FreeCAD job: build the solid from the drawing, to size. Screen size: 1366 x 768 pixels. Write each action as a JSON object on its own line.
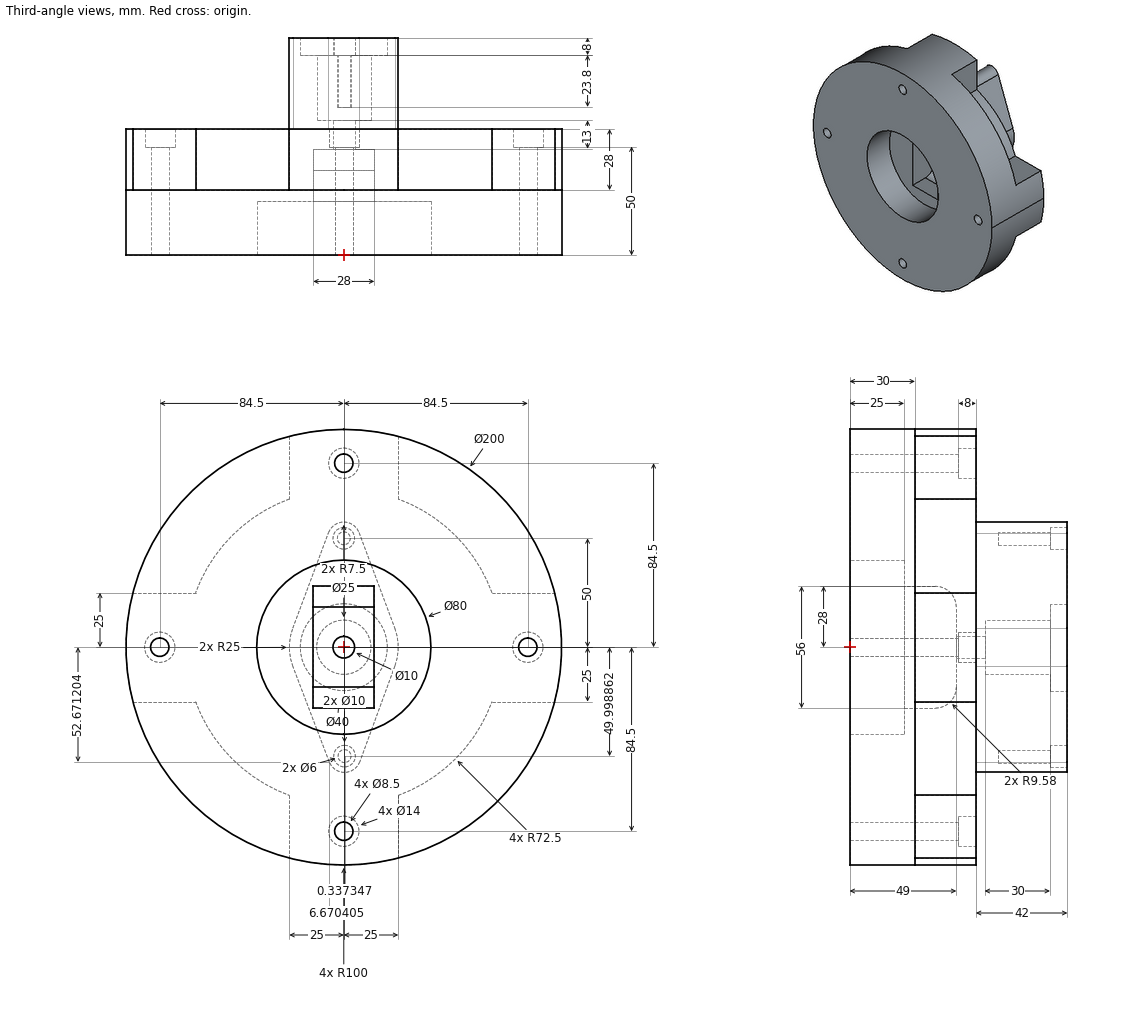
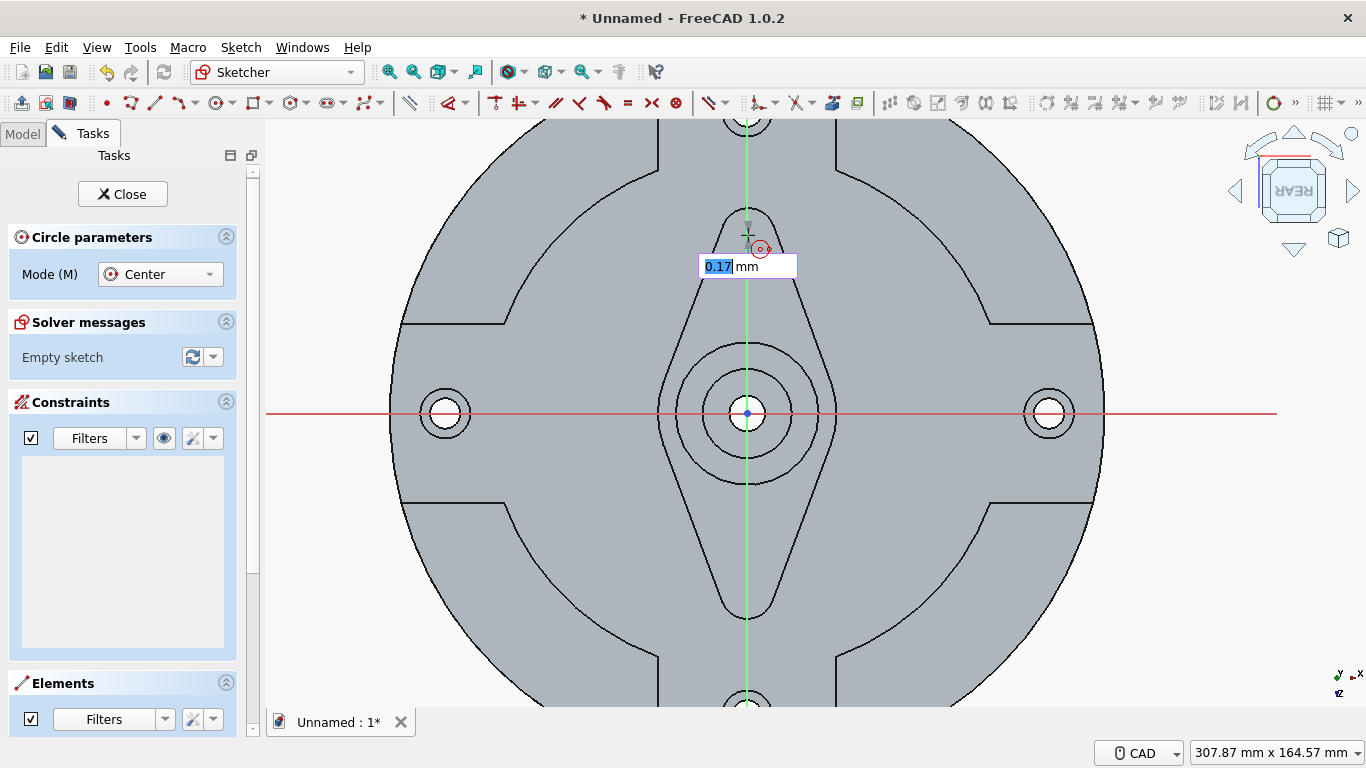
{"action": "left_click", "coordinate": [761, 222]}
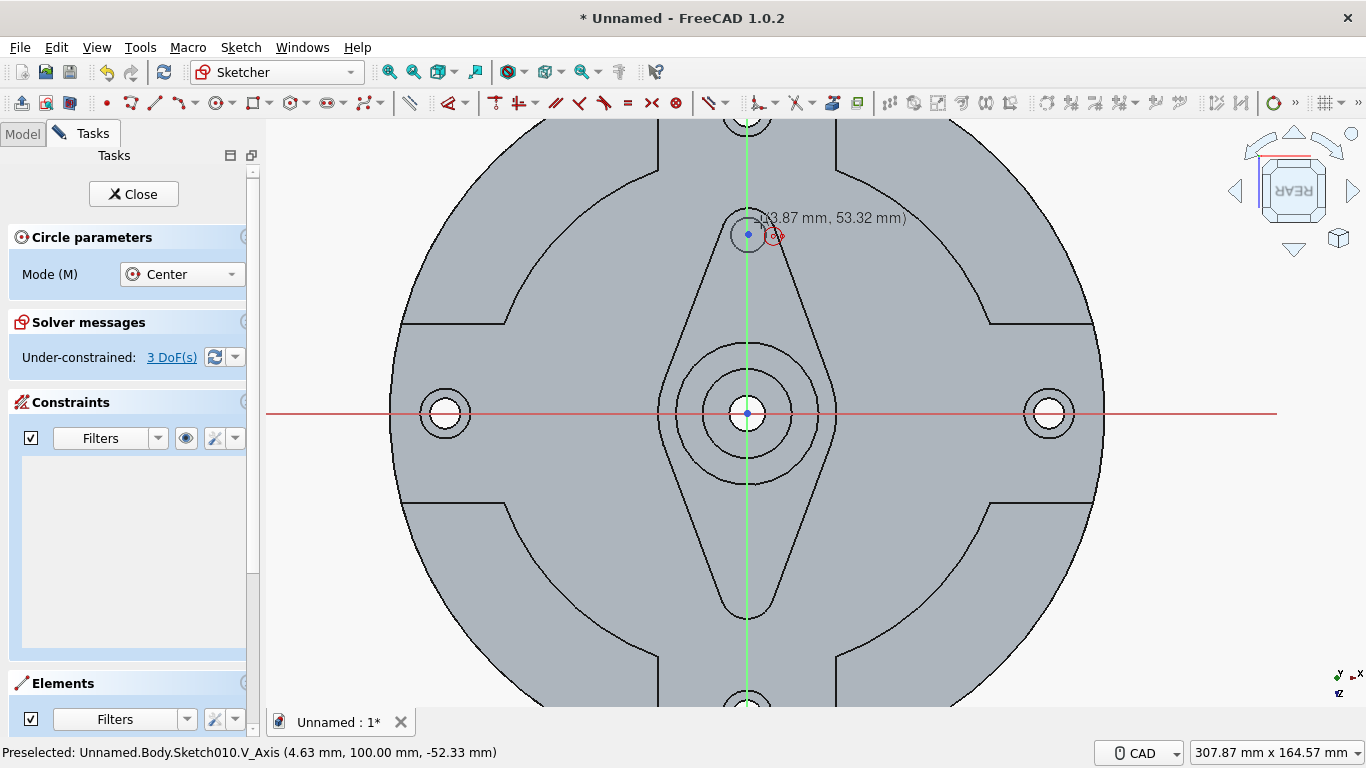
{"action": "scroll", "coordinate": [747, 592], "scroll_direction": "up", "scroll_amount": 2}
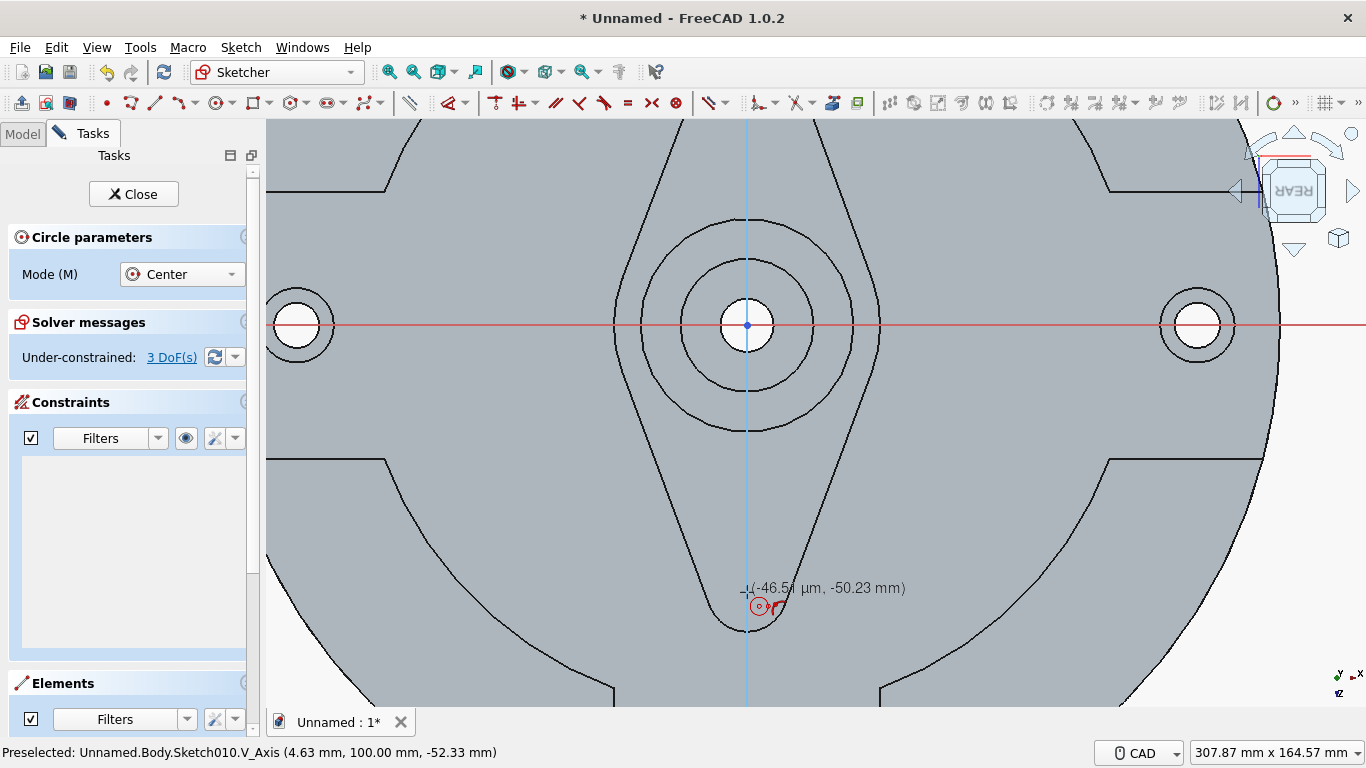
{"action": "left_click", "coordinate": [747, 592]}
{"action": "left_click", "coordinate": [766, 573]}
{"action": "key", "text": "Escape"}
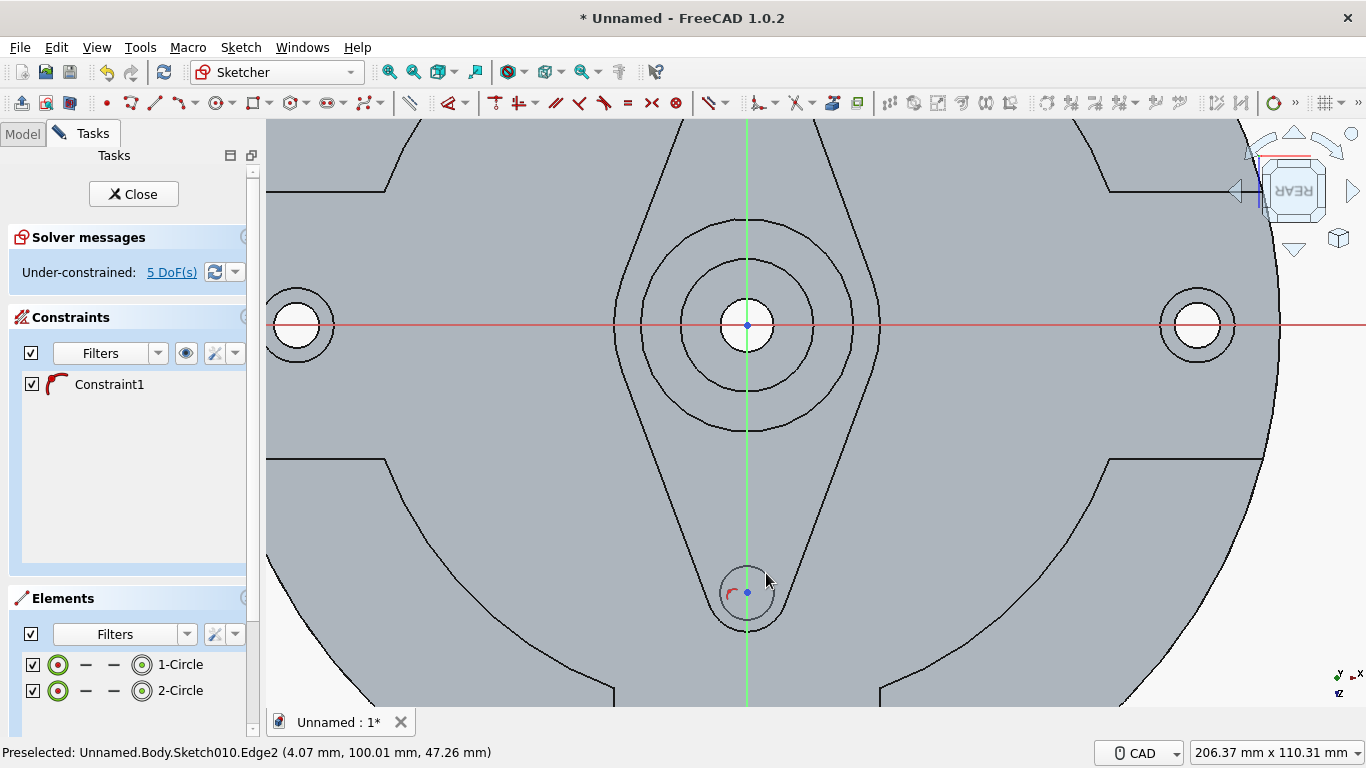
{"action": "scroll", "coordinate": [747, 591], "scroll_direction": "down", "scroll_amount": 2}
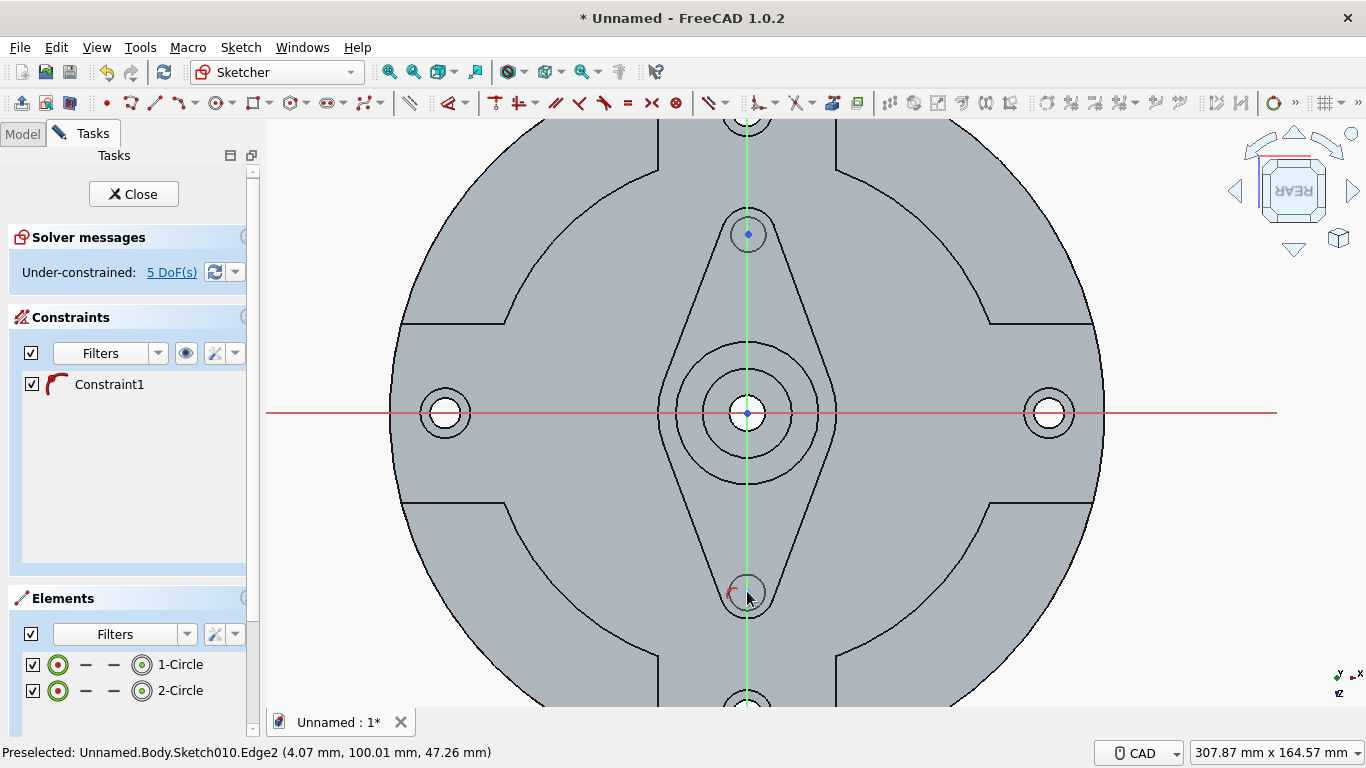
{"action": "left_click", "coordinate": [761, 222]}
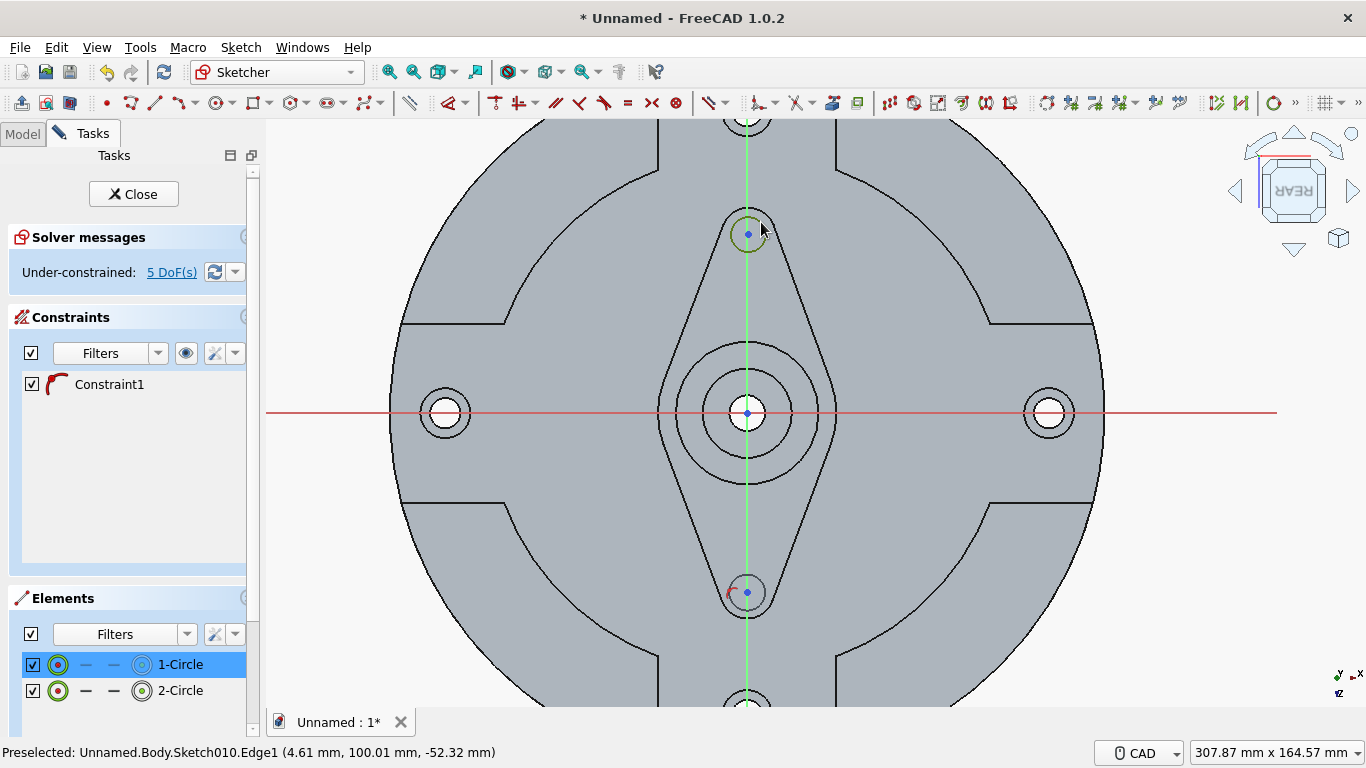
{"action": "left_click", "coordinate": [760, 580]}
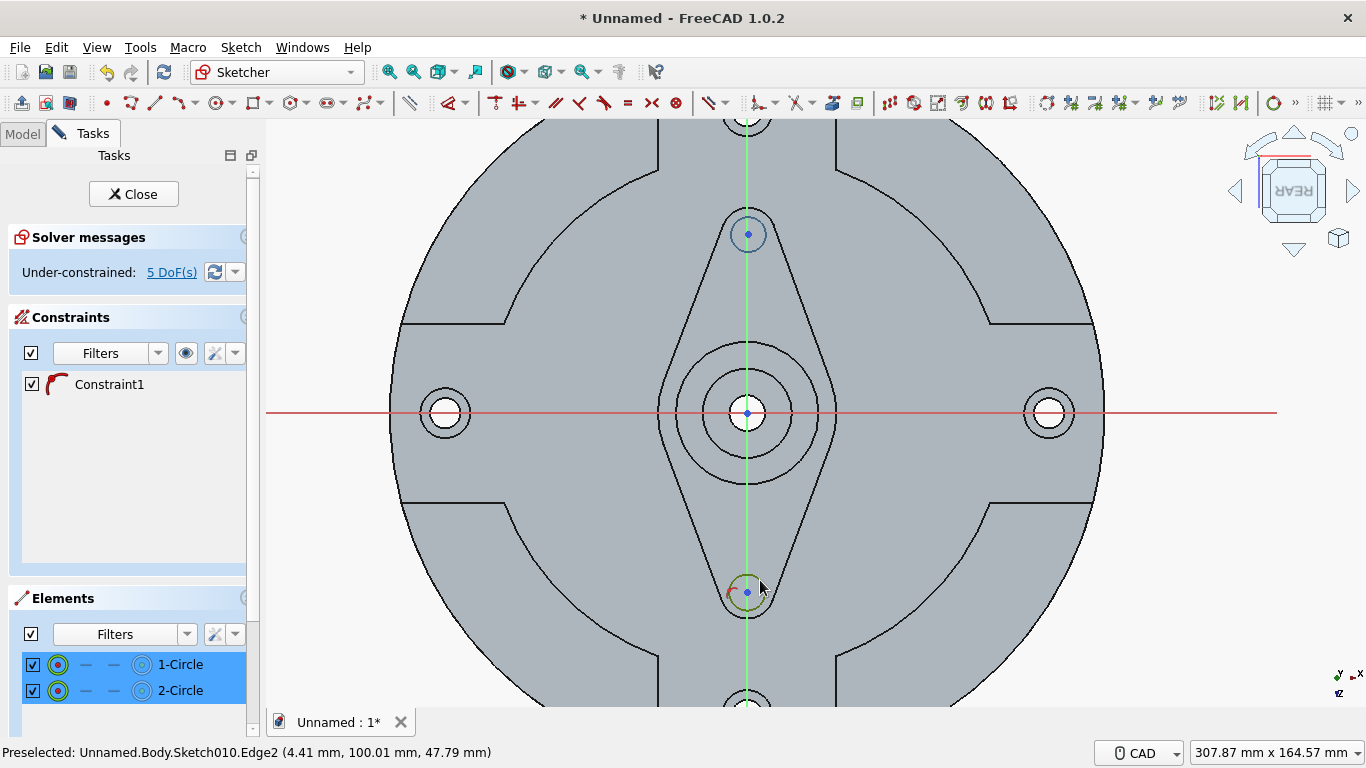
{"action": "key", "text": "e"}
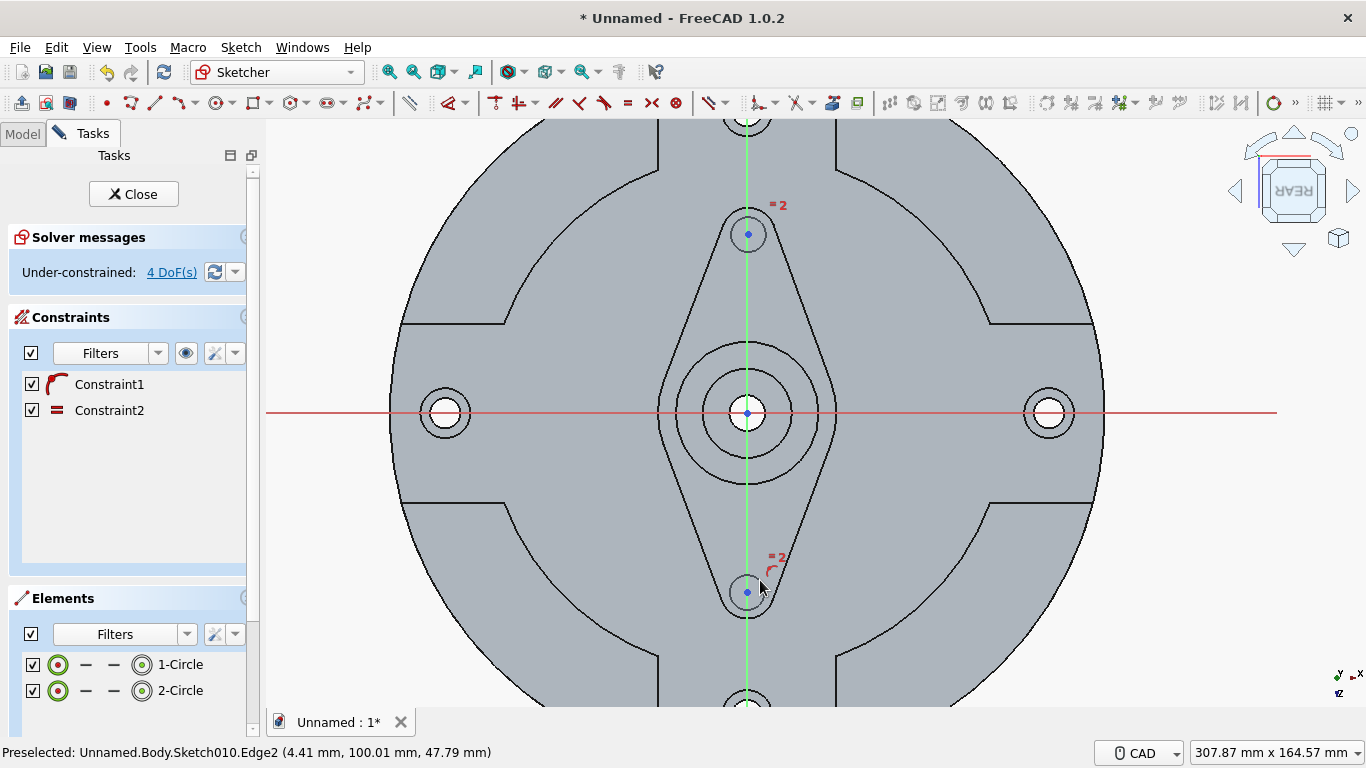
{"action": "key", "text": "d"}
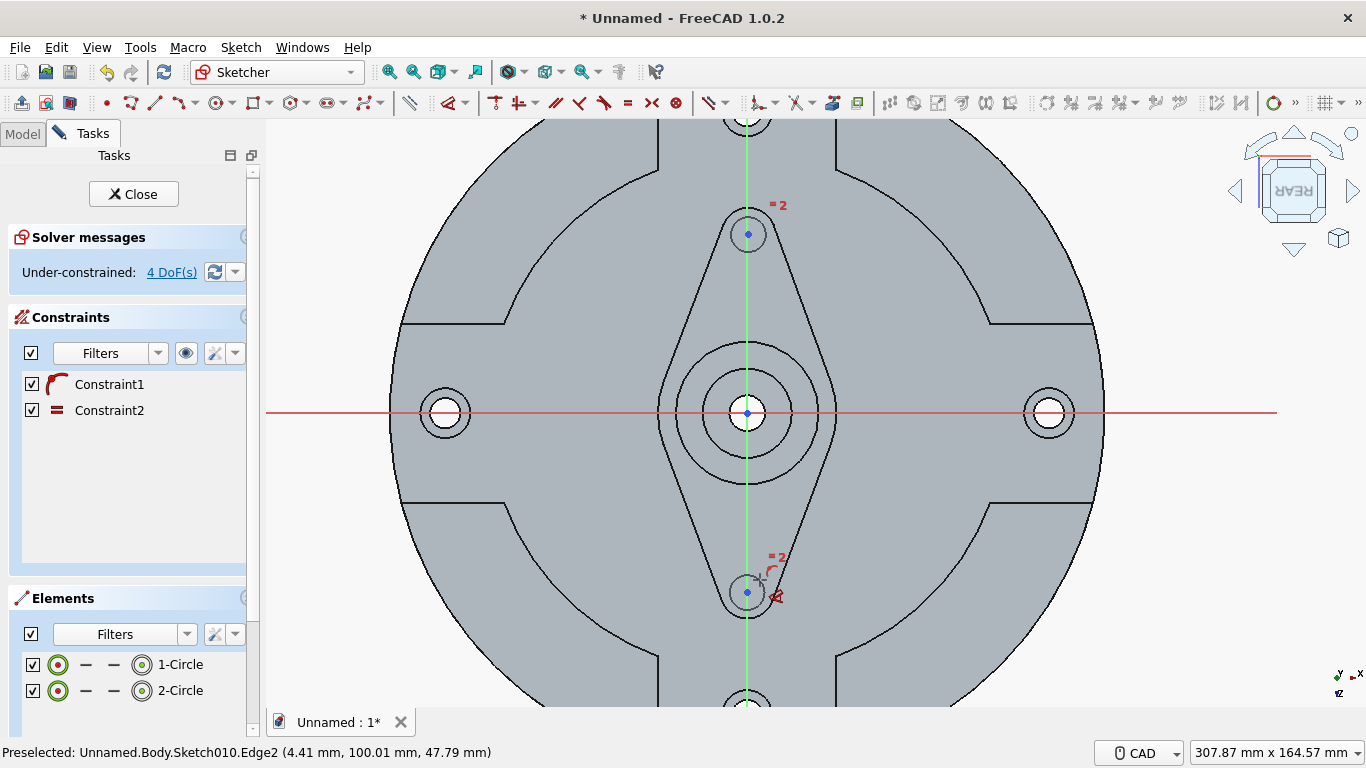
{"action": "left_click", "coordinate": [761, 222]}
{"action": "left_click", "coordinate": [784, 199]}